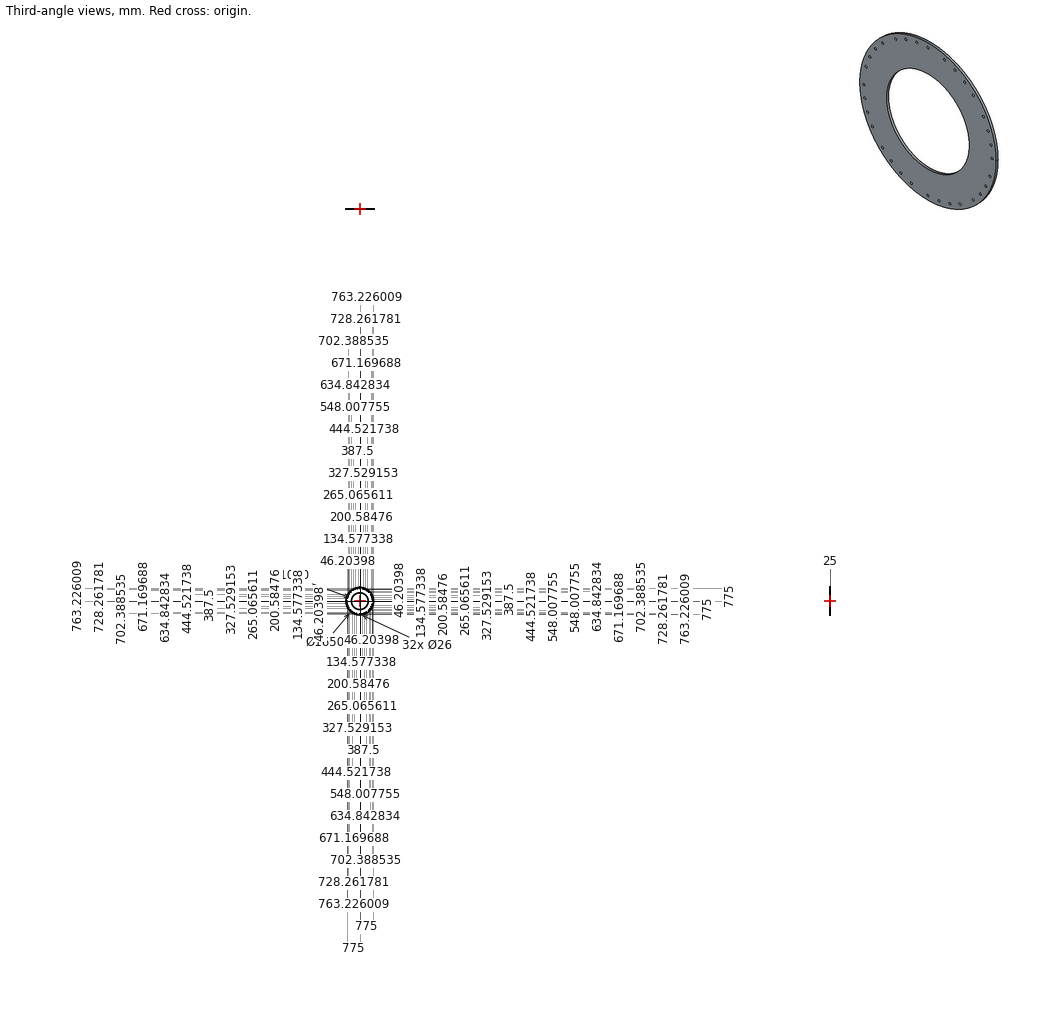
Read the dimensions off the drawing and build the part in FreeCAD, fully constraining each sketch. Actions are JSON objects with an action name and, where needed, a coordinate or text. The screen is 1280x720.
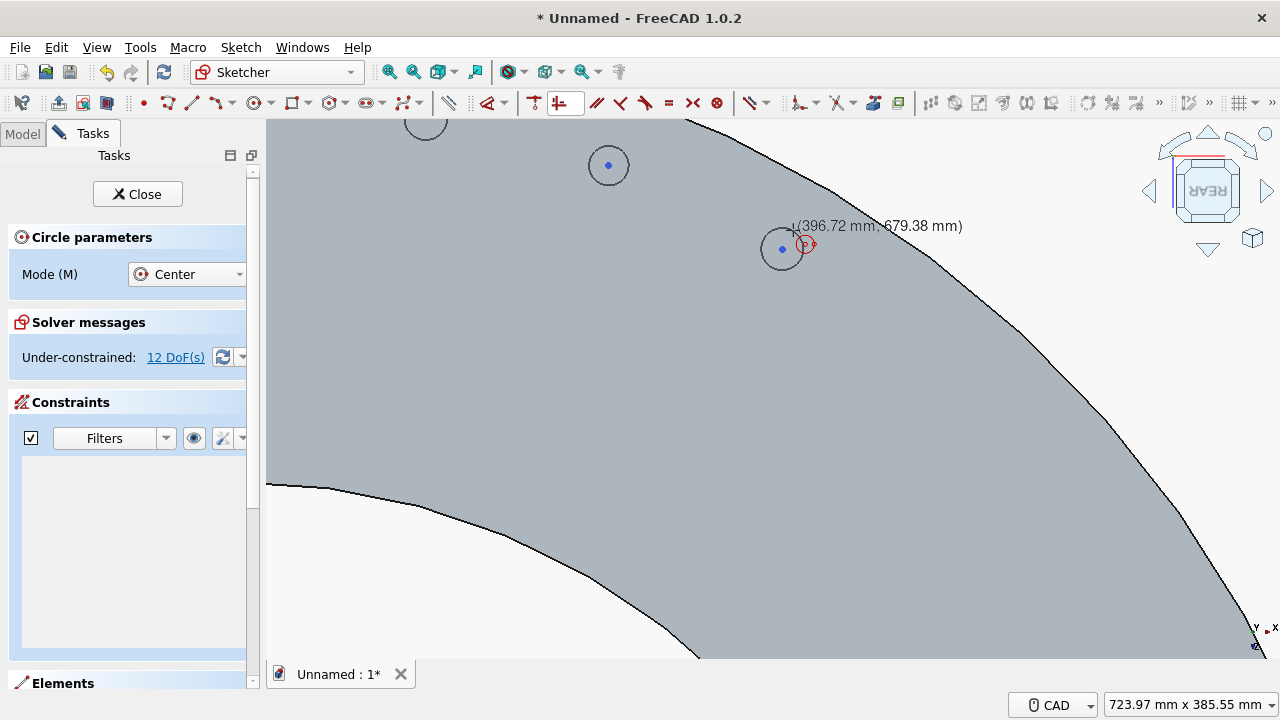
{"action": "scroll", "coordinate": [1005, 415], "scroll_direction": "up", "scroll_amount": 2}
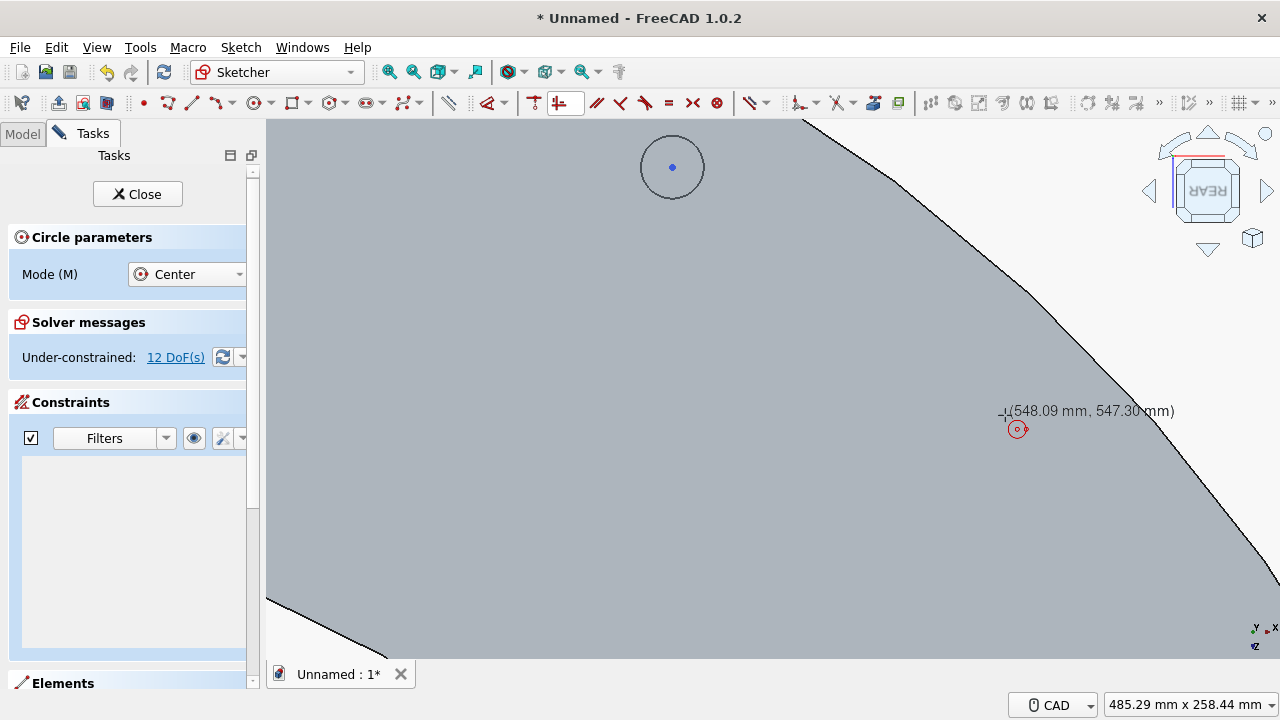
{"action": "scroll", "coordinate": [810, 243], "scroll_direction": "down", "scroll_amount": 11}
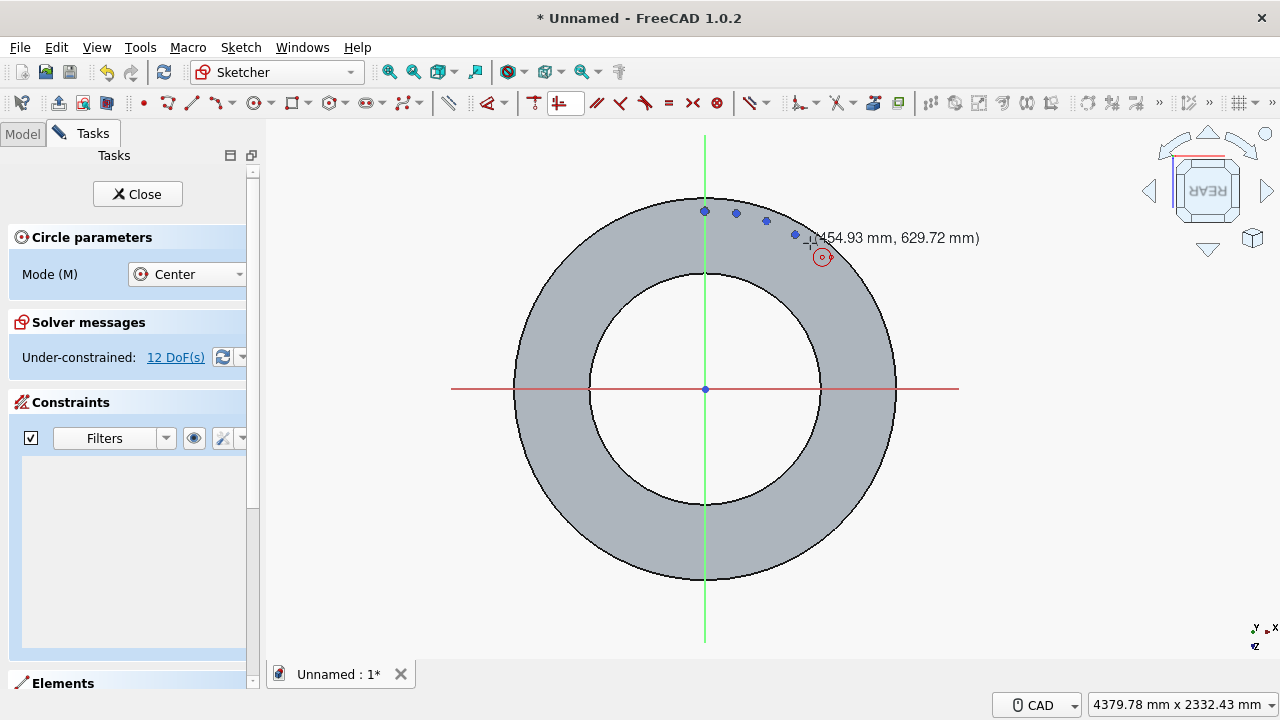
{"action": "left_click", "coordinate": [832, 262]}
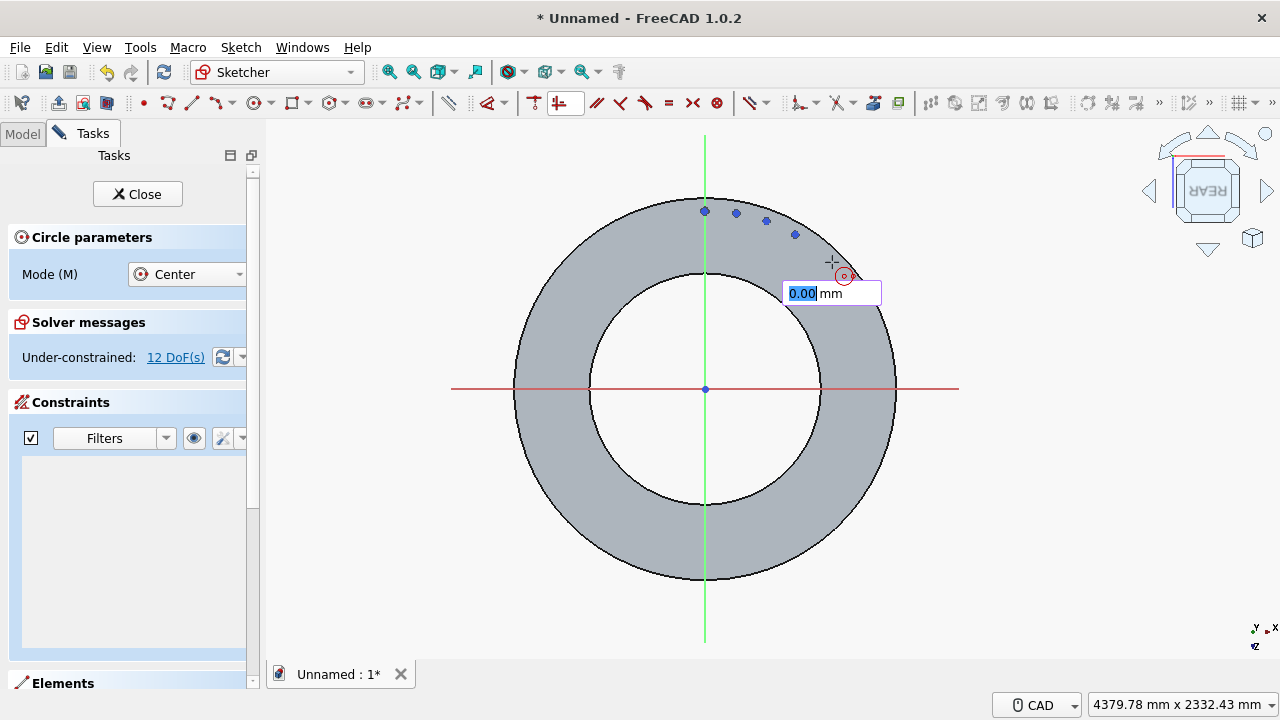
{"action": "scroll", "coordinate": [834, 260], "scroll_direction": "up", "scroll_amount": 9}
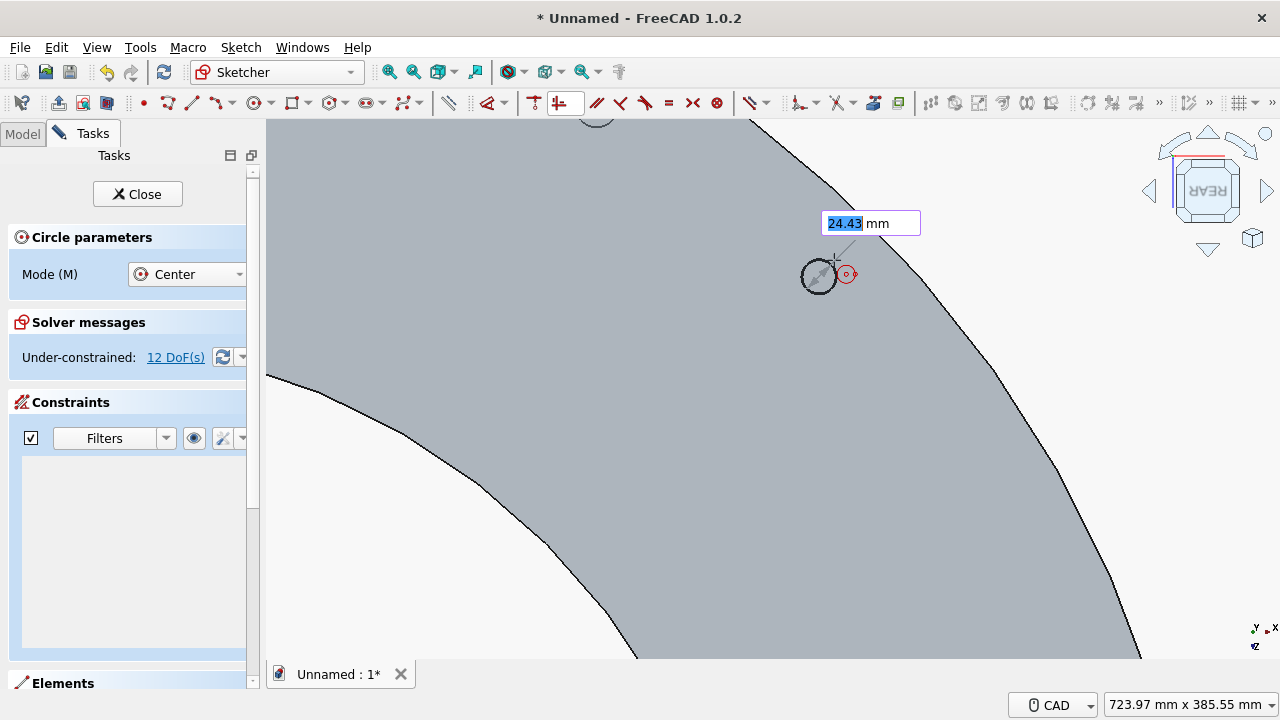
{"action": "left_click", "coordinate": [832, 259]}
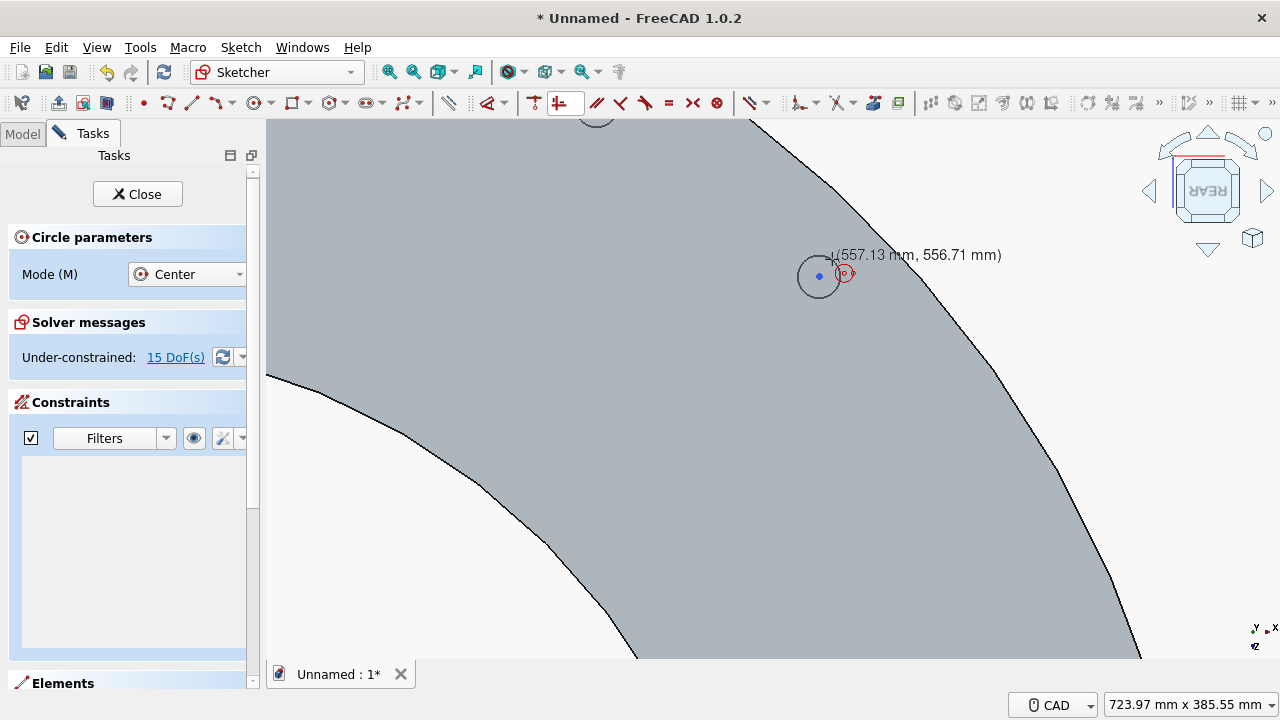
{"action": "scroll", "coordinate": [941, 417], "scroll_direction": "up", "scroll_amount": 2}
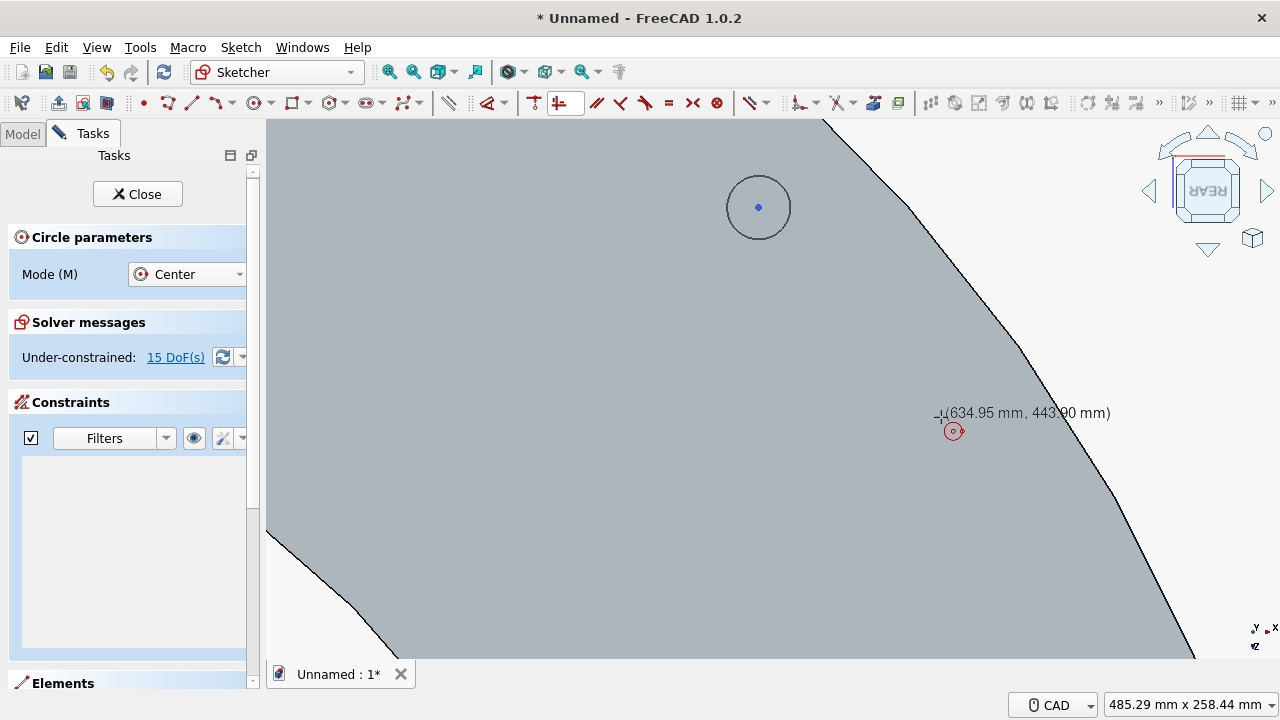
{"action": "scroll", "coordinate": [840, 270], "scroll_direction": "down", "scroll_amount": 11}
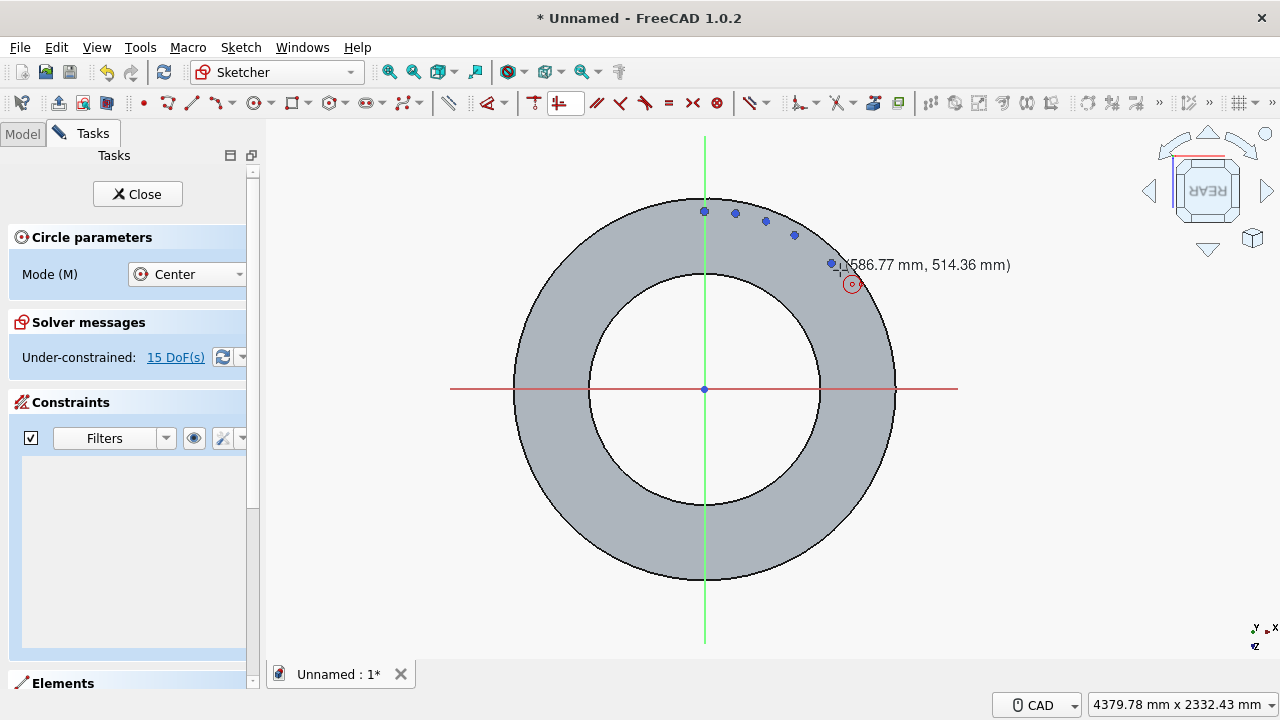
{"action": "left_click", "coordinate": [852, 287]}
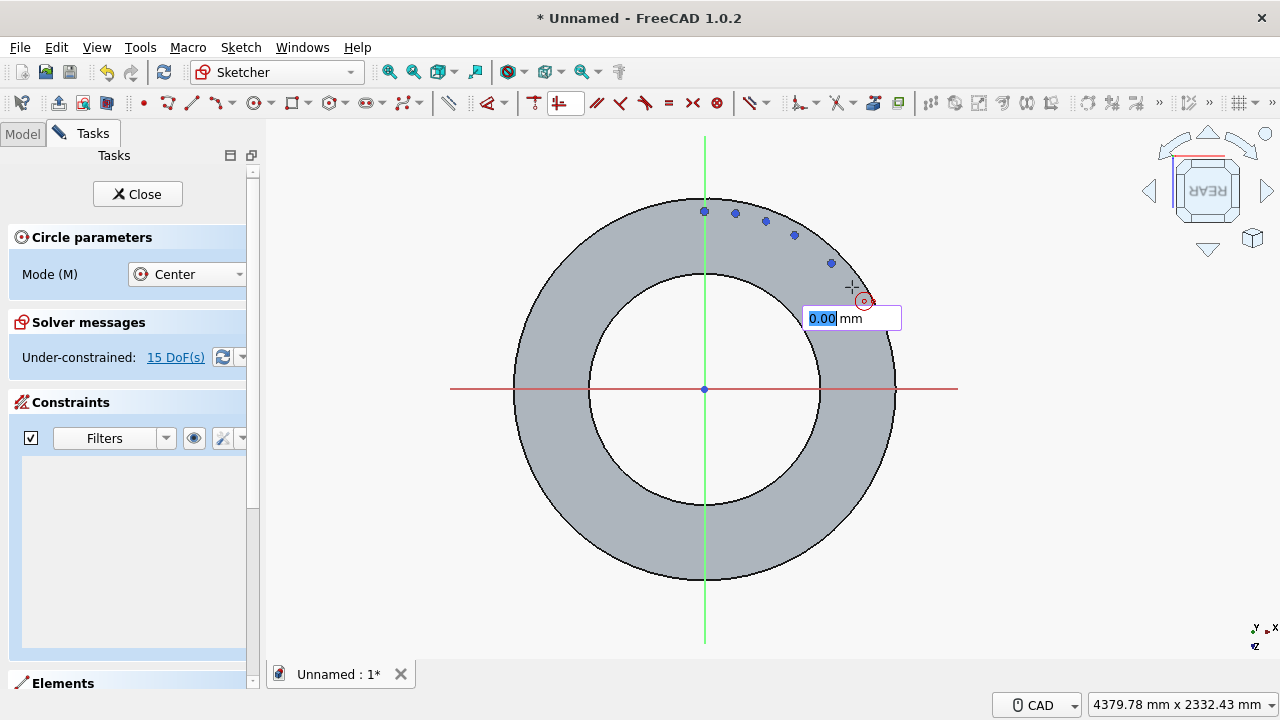
{"action": "scroll", "coordinate": [854, 284], "scroll_direction": "up", "scroll_amount": 9}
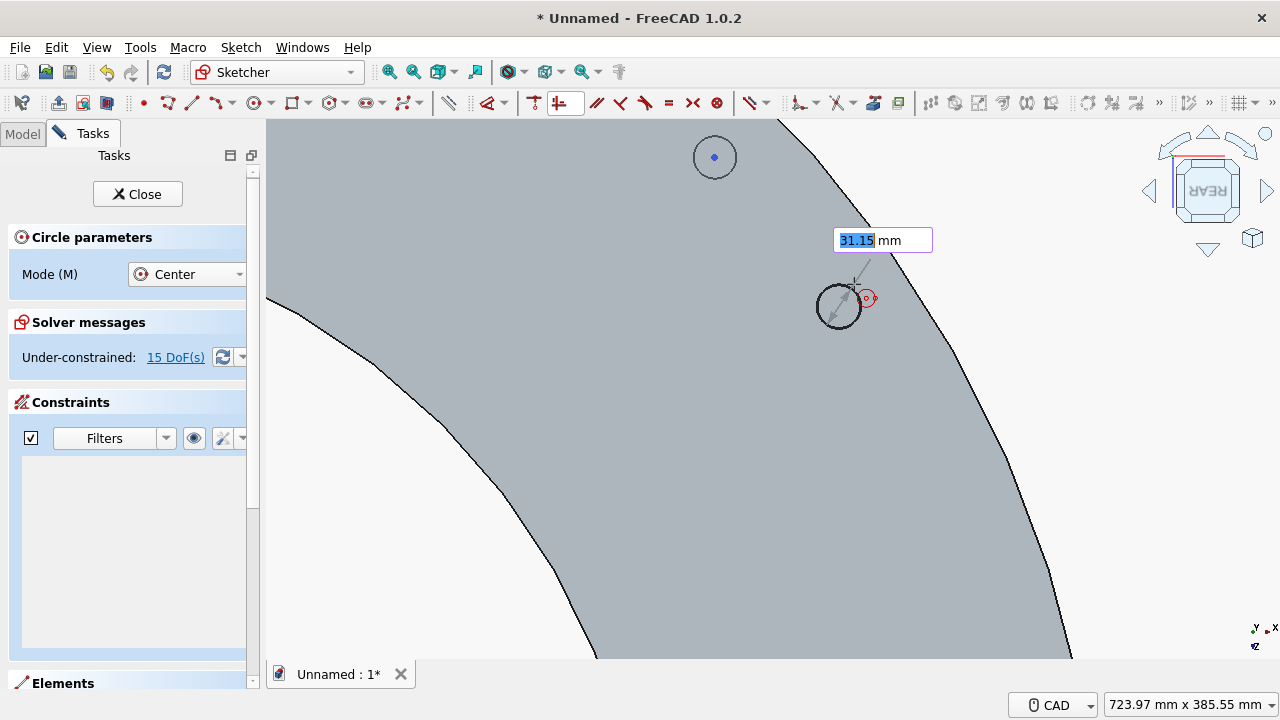
{"action": "left_click", "coordinate": [850, 285]}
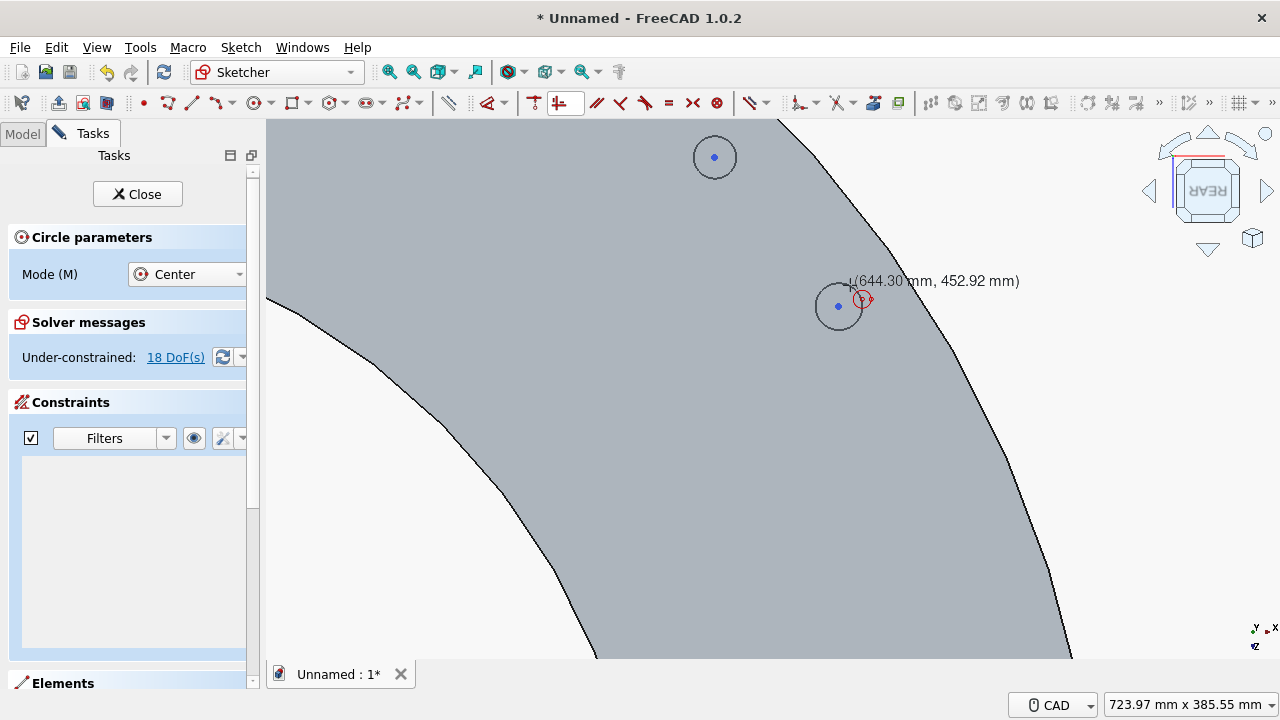
{"action": "scroll", "coordinate": [931, 462], "scroll_direction": "up", "scroll_amount": 2}